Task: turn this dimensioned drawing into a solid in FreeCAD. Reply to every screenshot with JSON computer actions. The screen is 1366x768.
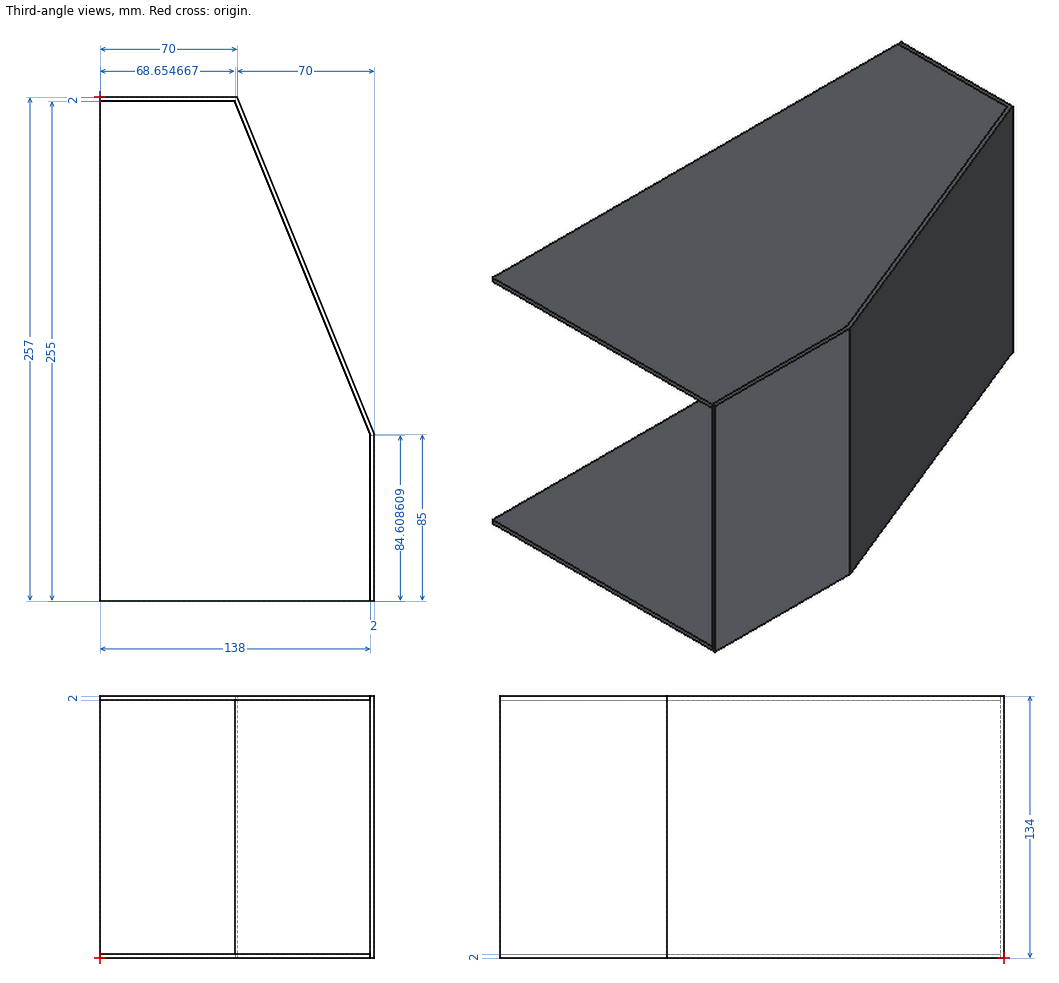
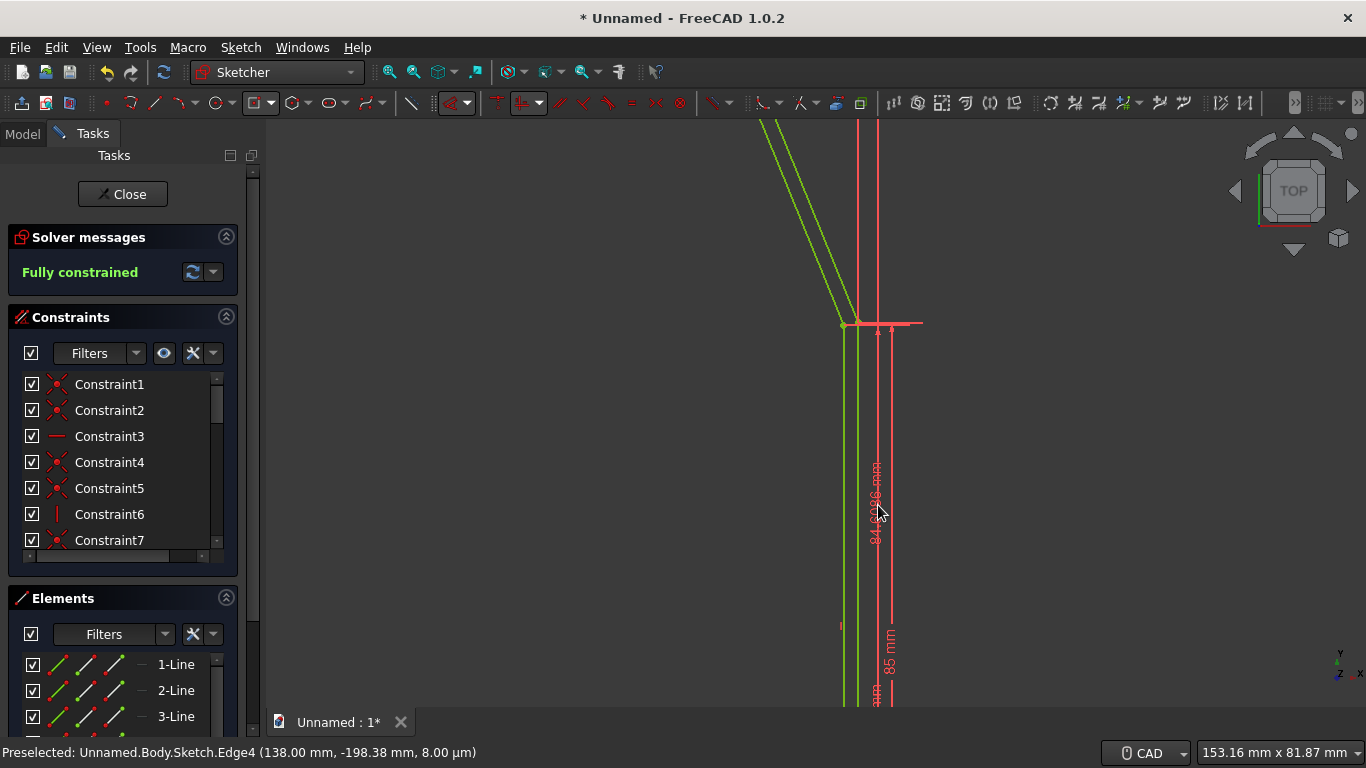
{"action": "left_click", "coordinate": [123, 194]}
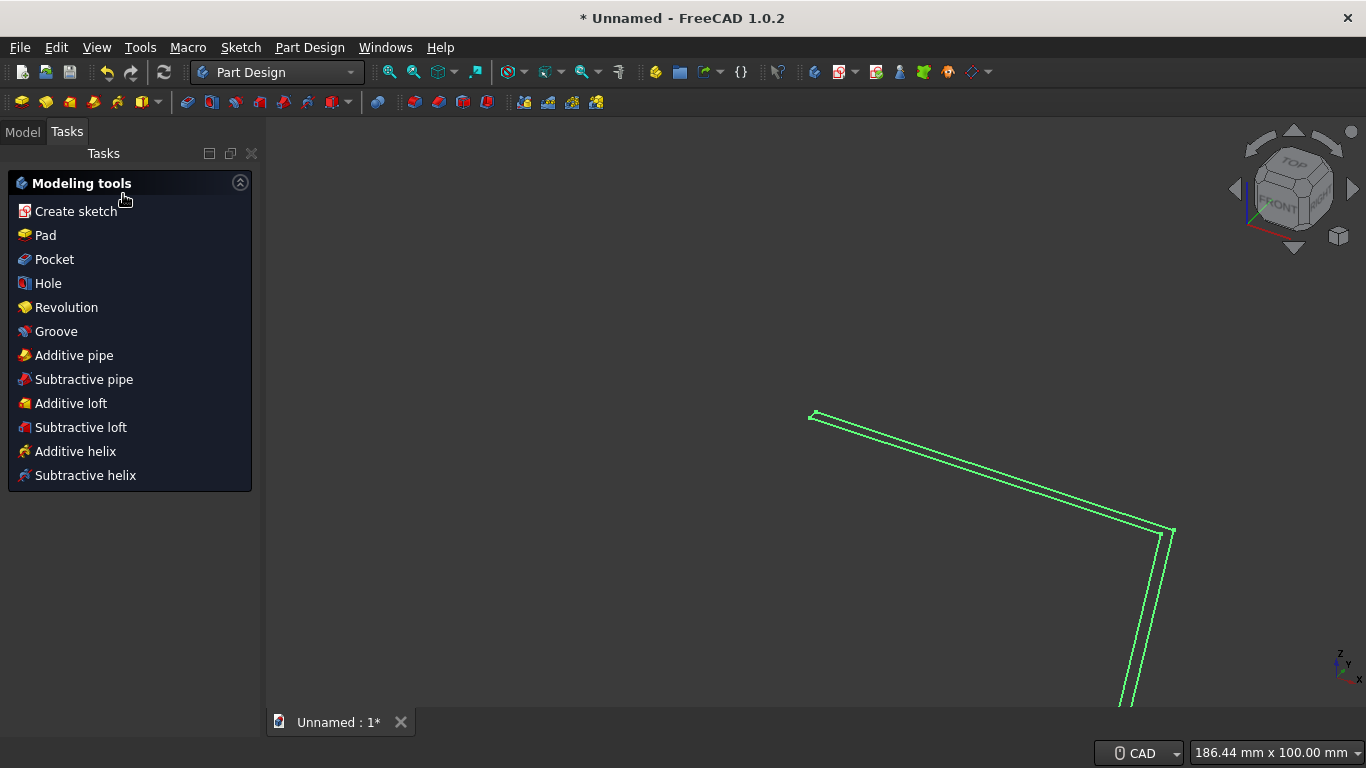
{"action": "left_click", "coordinate": [22, 102]}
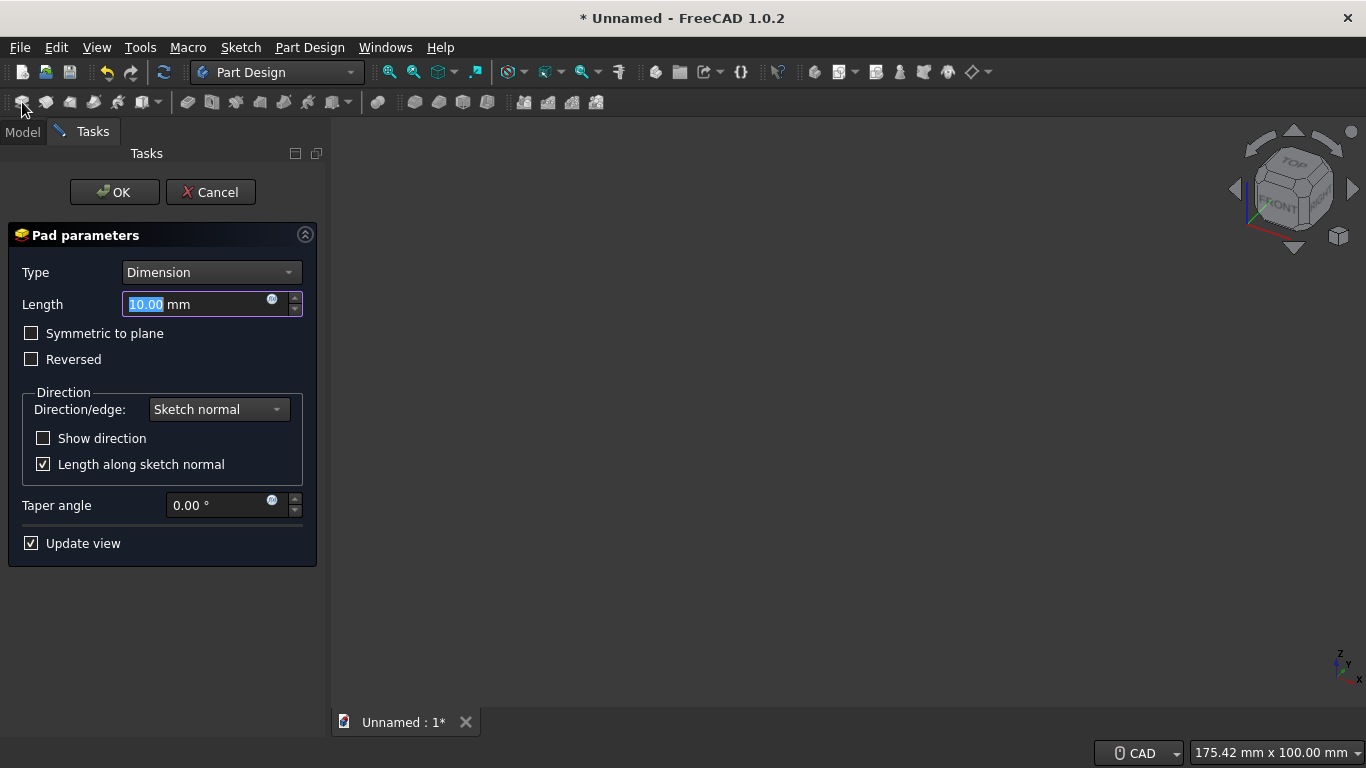
{"action": "type", "text": "134"}
{"action": "key", "text": "Tab"}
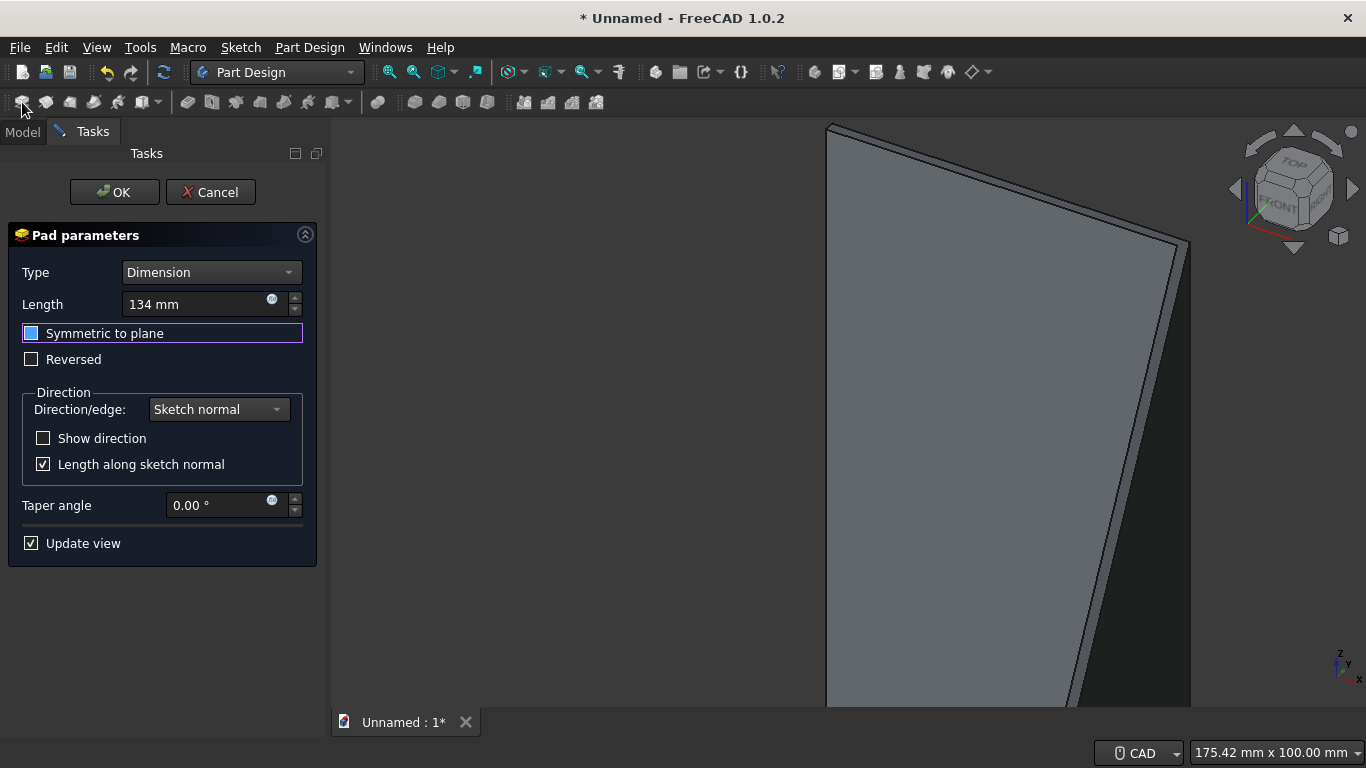
{"action": "left_click", "coordinate": [115, 192]}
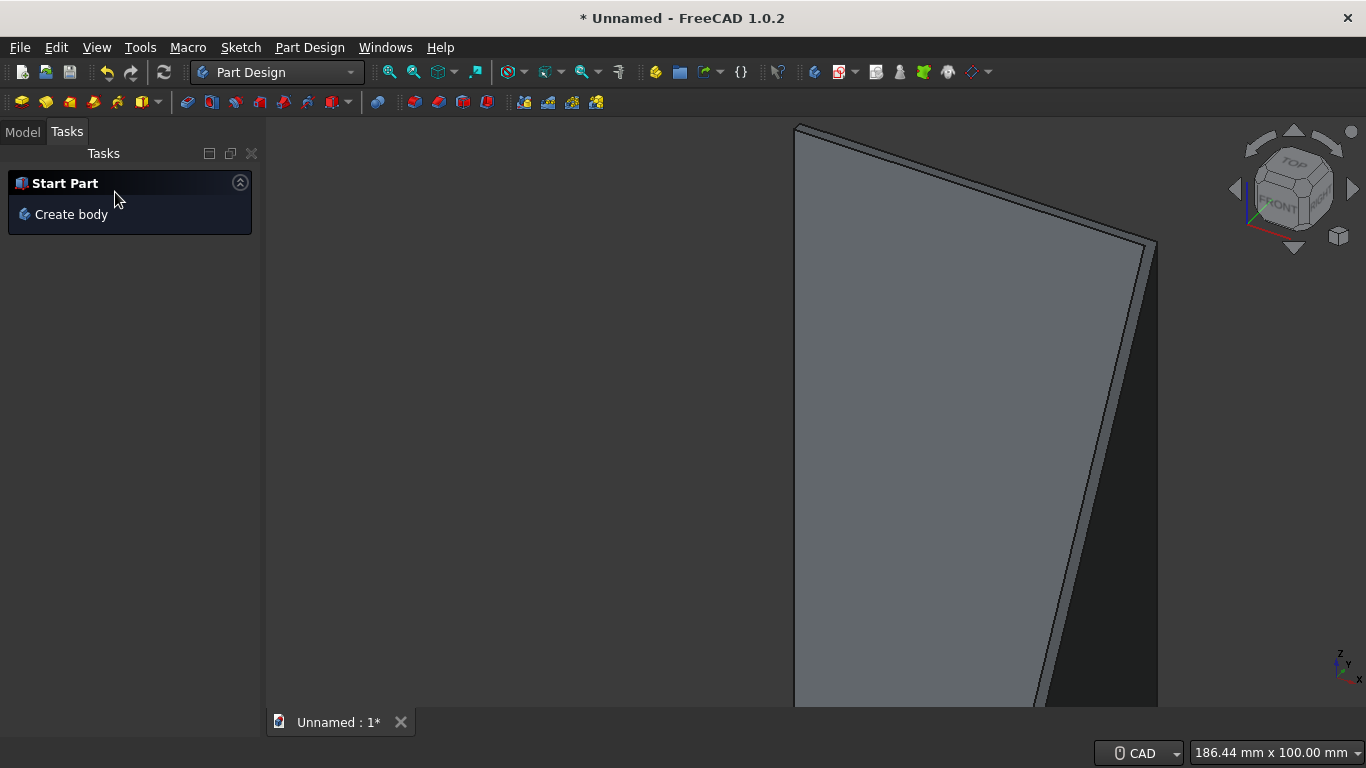
{"action": "key", "text": "v f"}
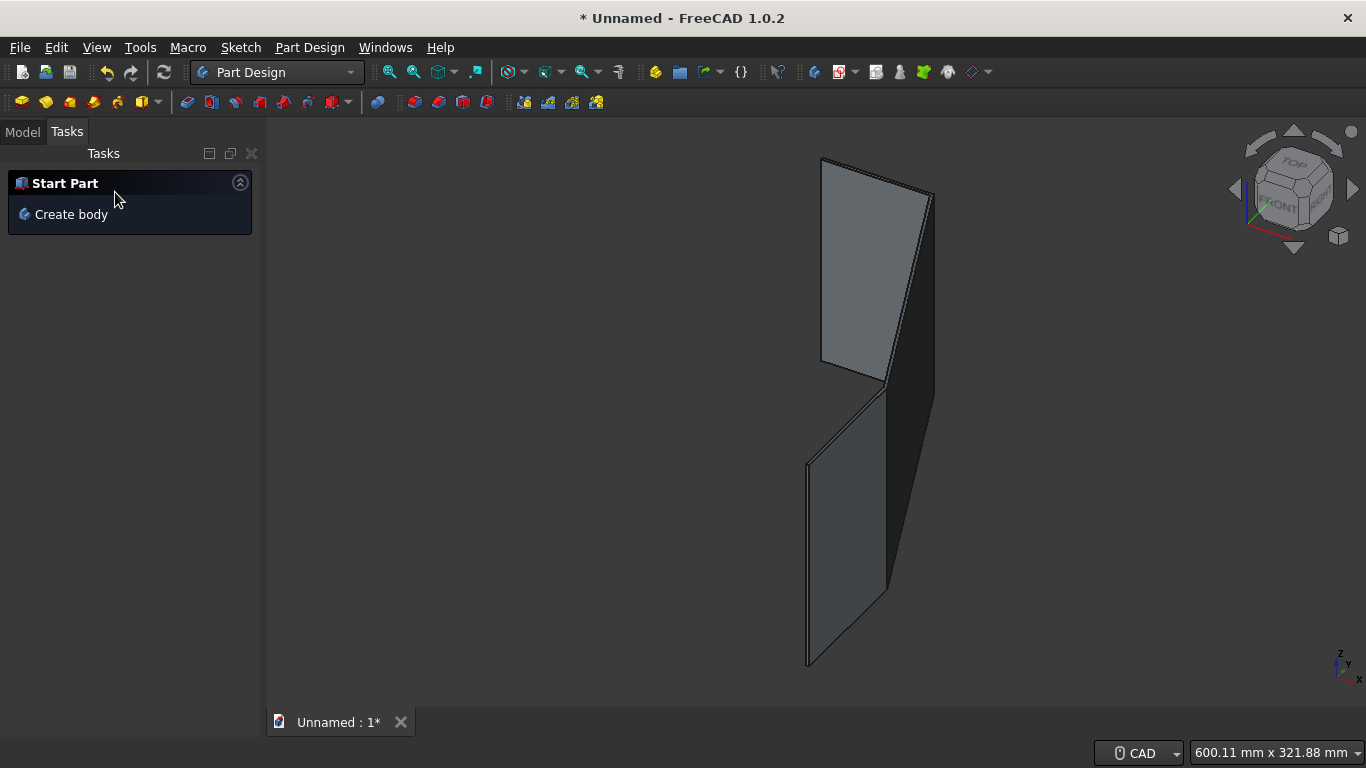
{"action": "left_click", "coordinate": [816, 72]}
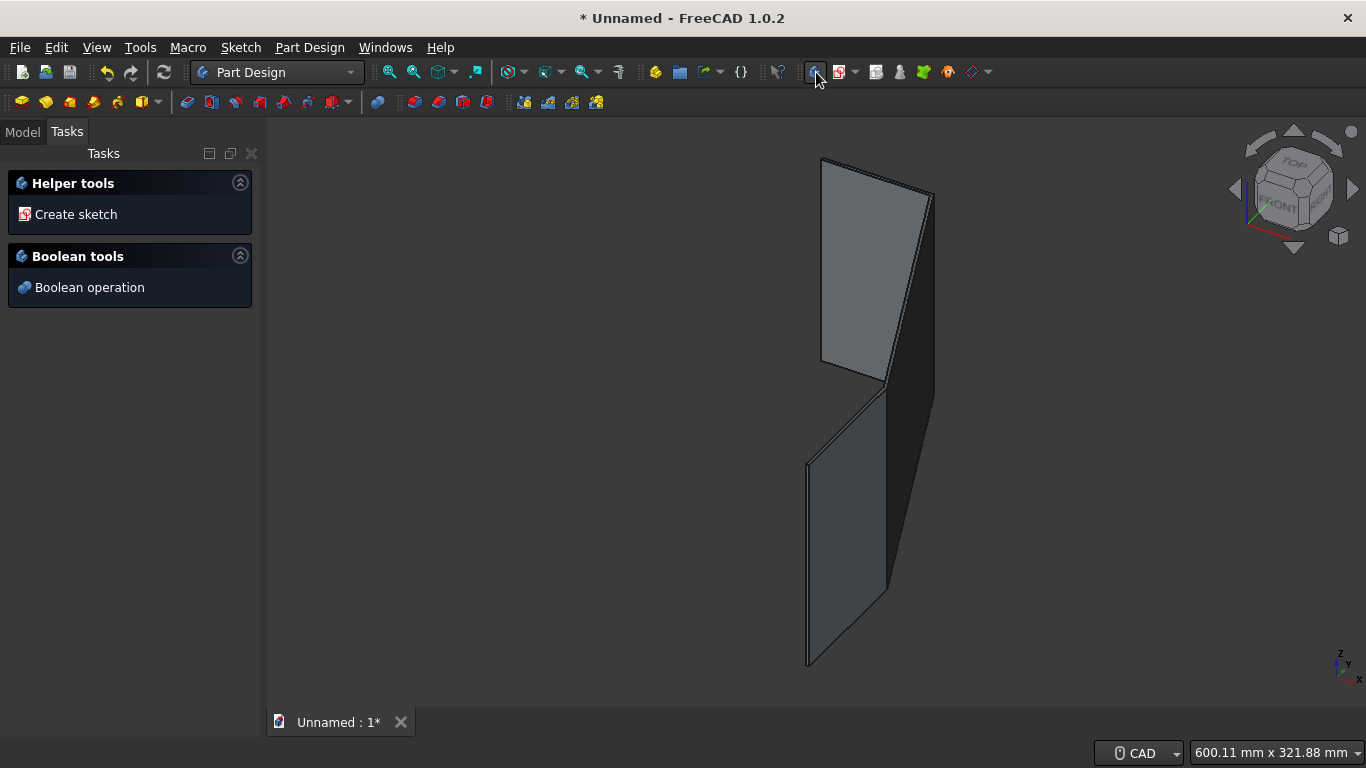
{"action": "left_click", "coordinate": [23, 131]}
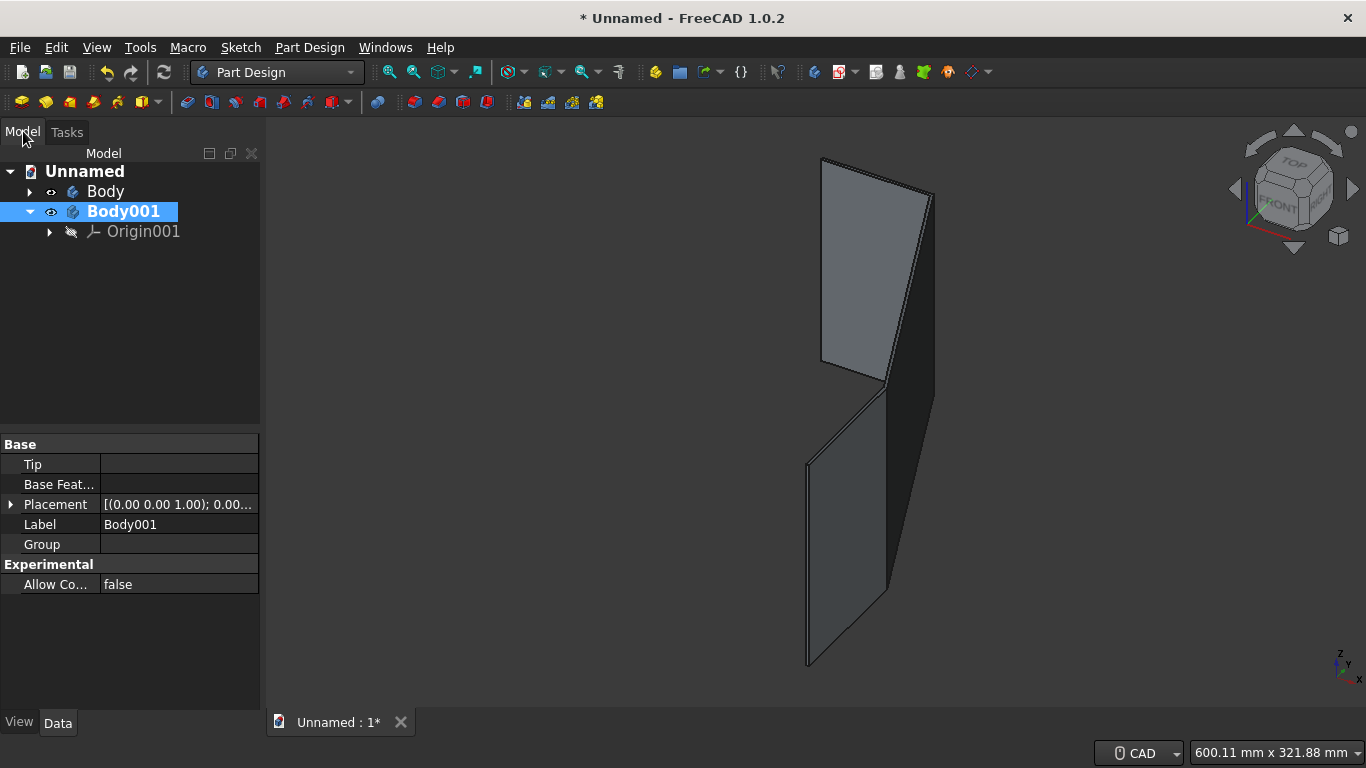
{"action": "left_click", "coordinate": [50, 232]}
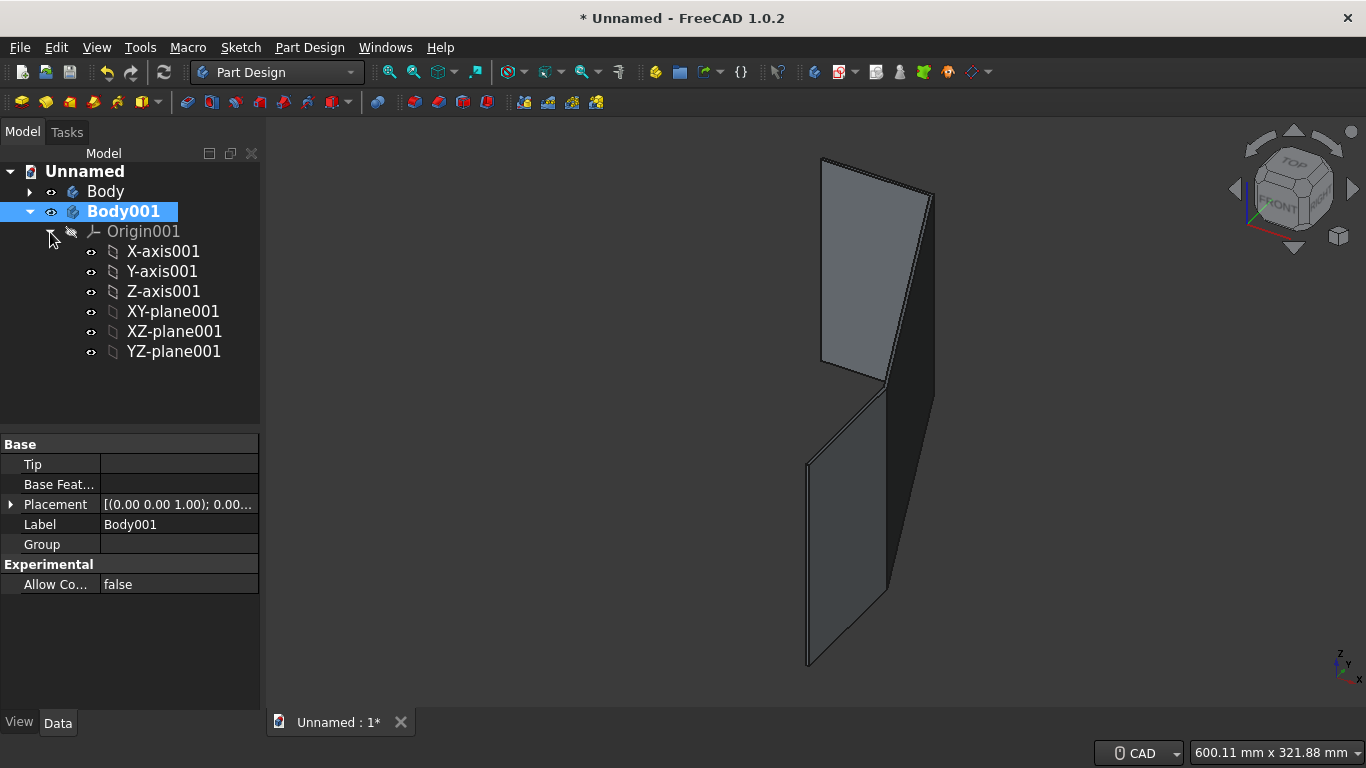
{"action": "left_click", "coordinate": [136, 312]}